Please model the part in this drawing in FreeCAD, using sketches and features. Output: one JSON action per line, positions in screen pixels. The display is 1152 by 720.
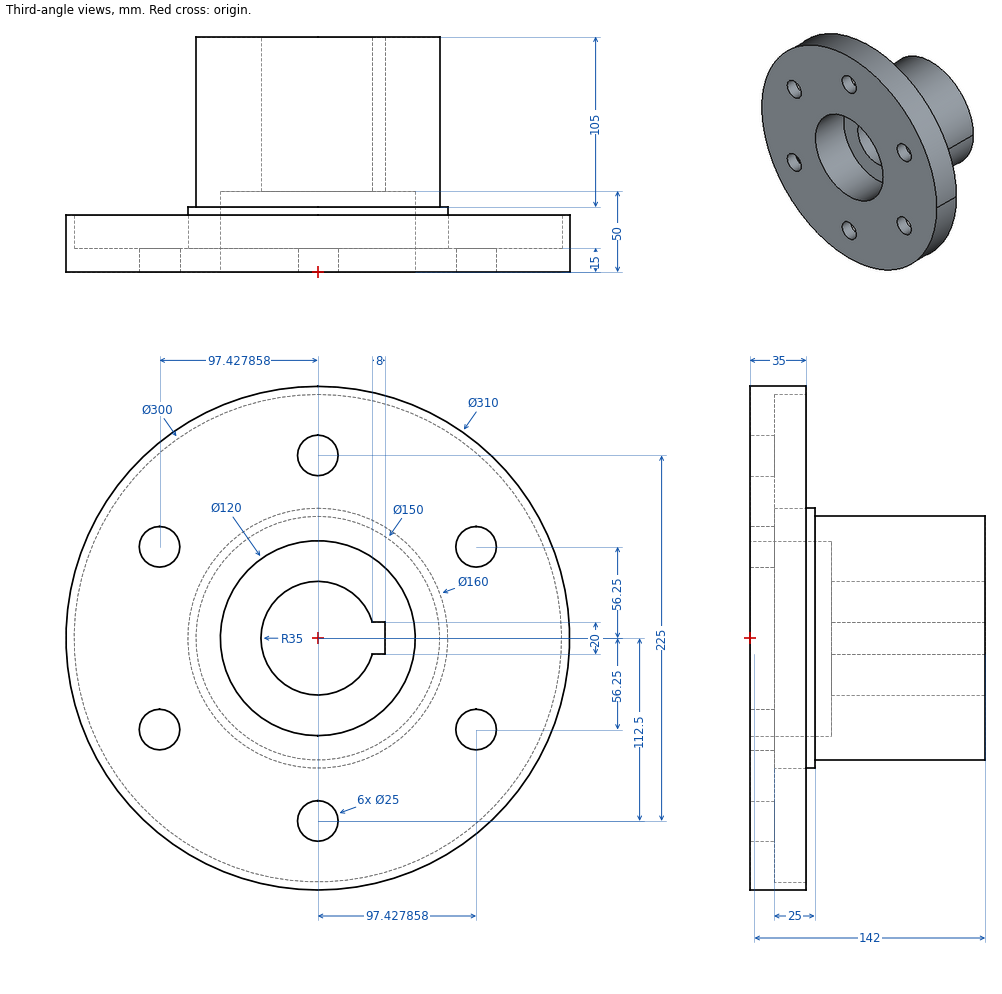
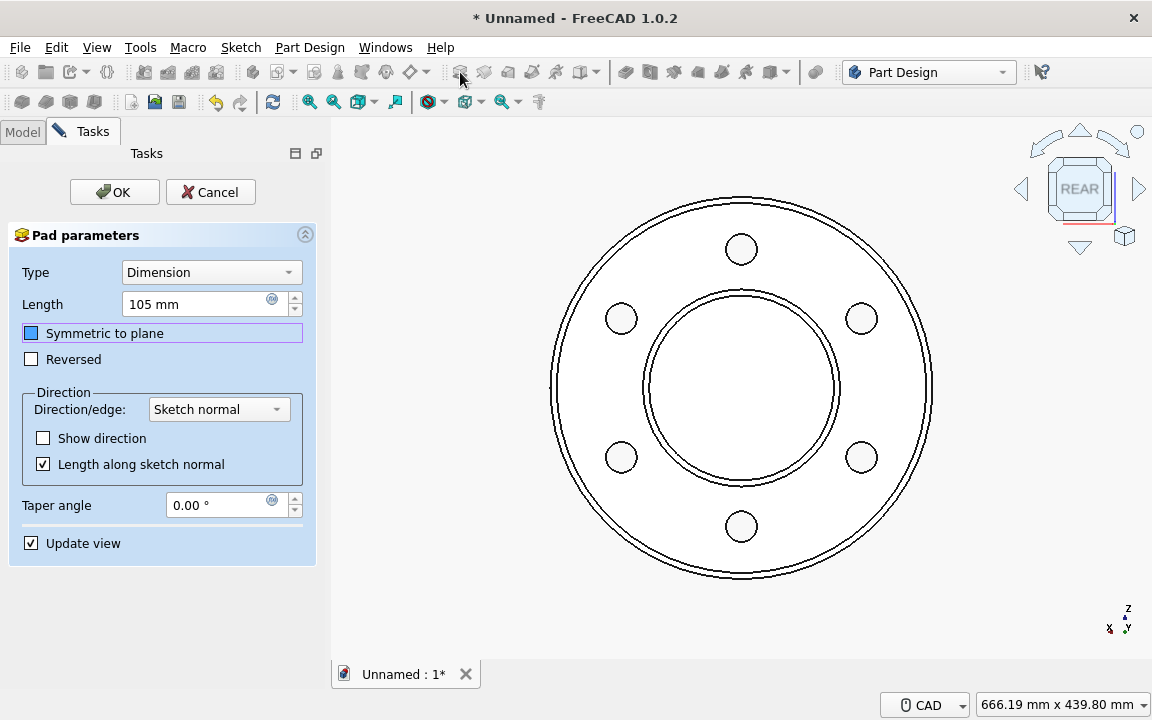
{"action": "left_click", "coordinate": [115, 192]}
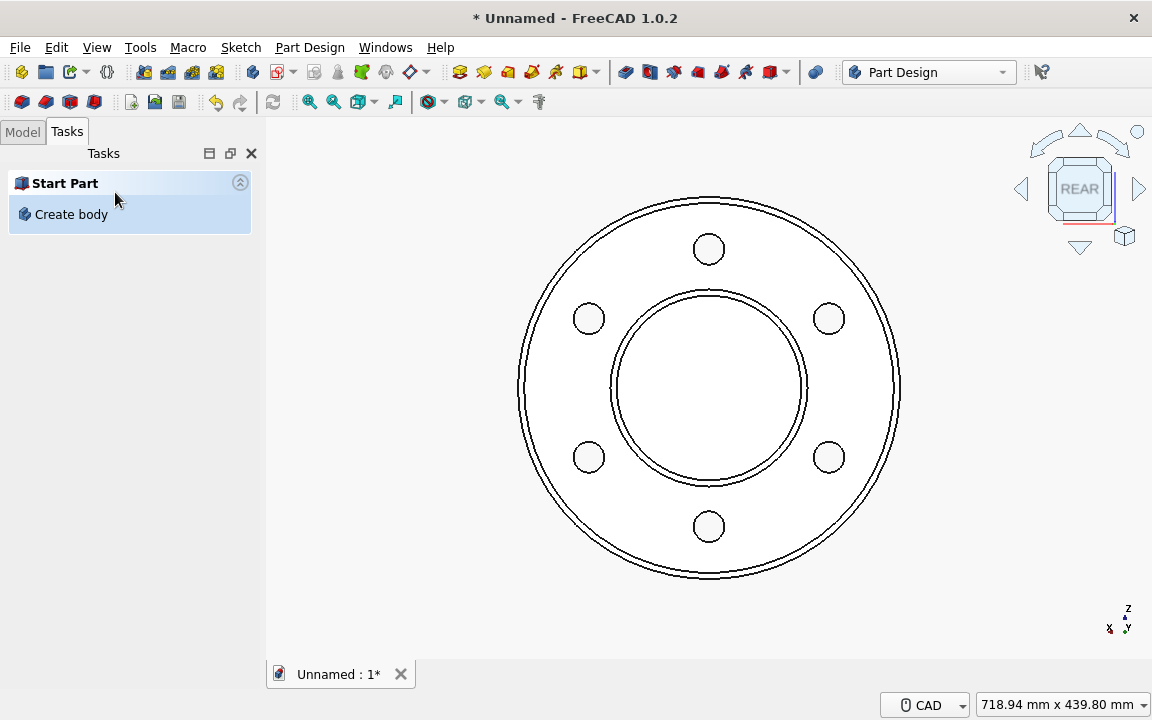
{"action": "left_click", "coordinate": [709, 387]}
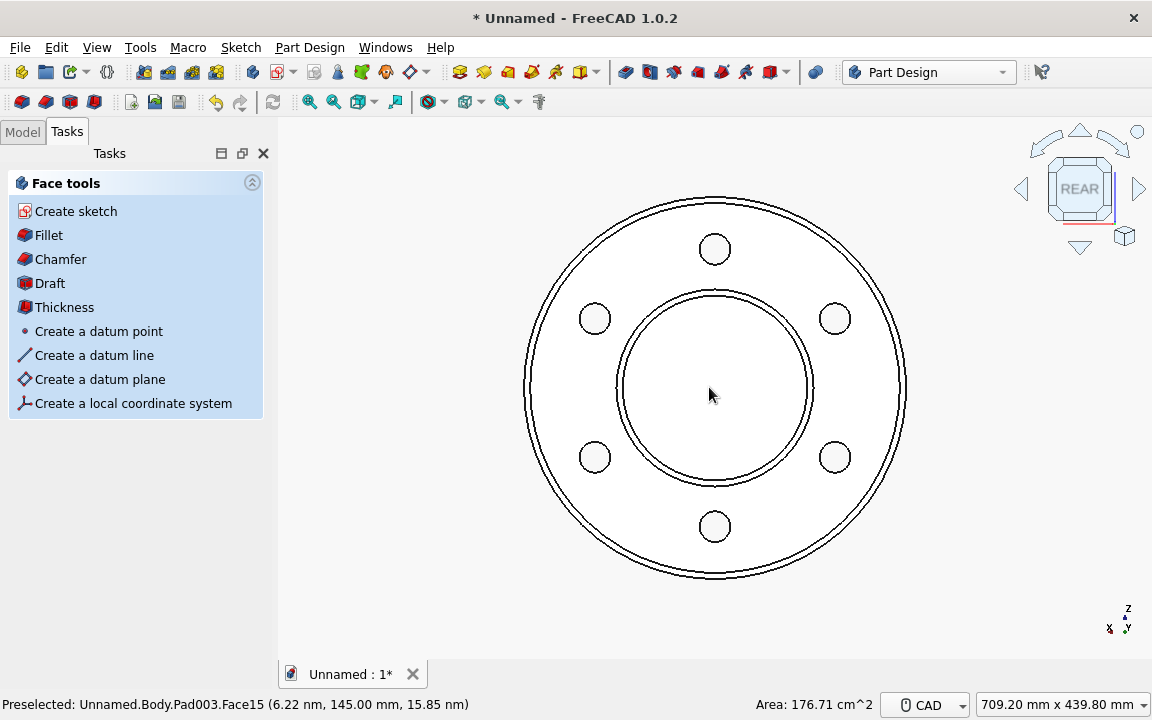
{"action": "left_click", "coordinate": [278, 72]}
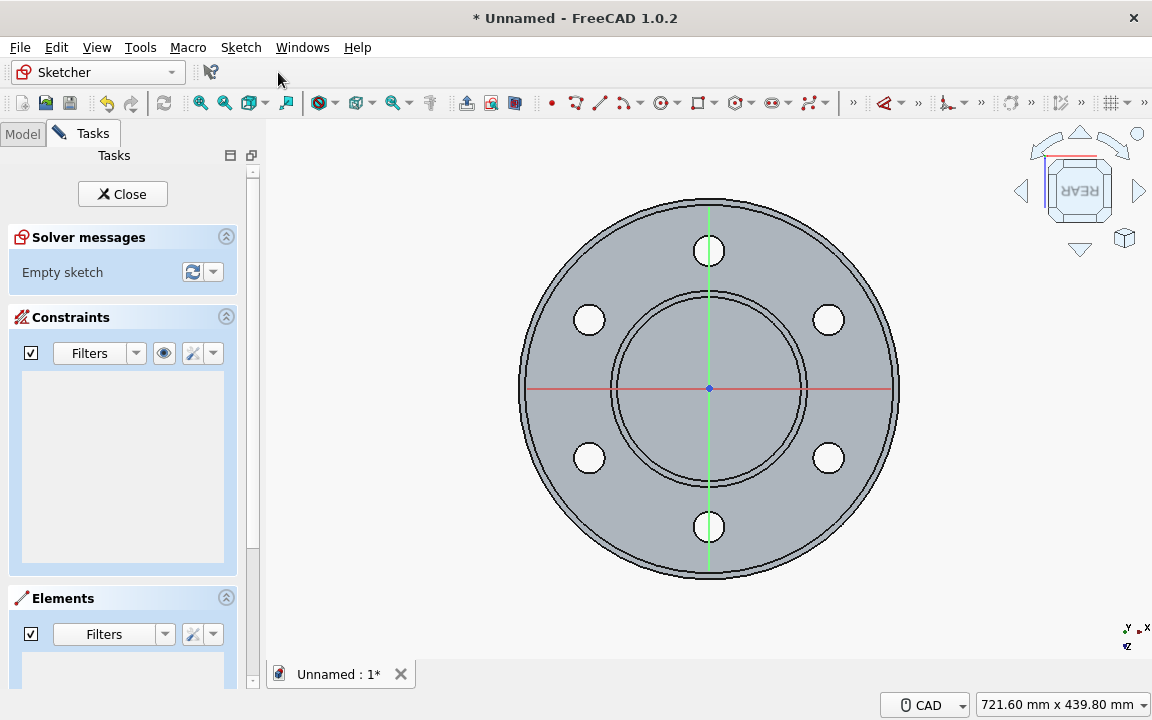
{"action": "scroll", "coordinate": [731, 389], "scroll_direction": "up", "scroll_amount": 8}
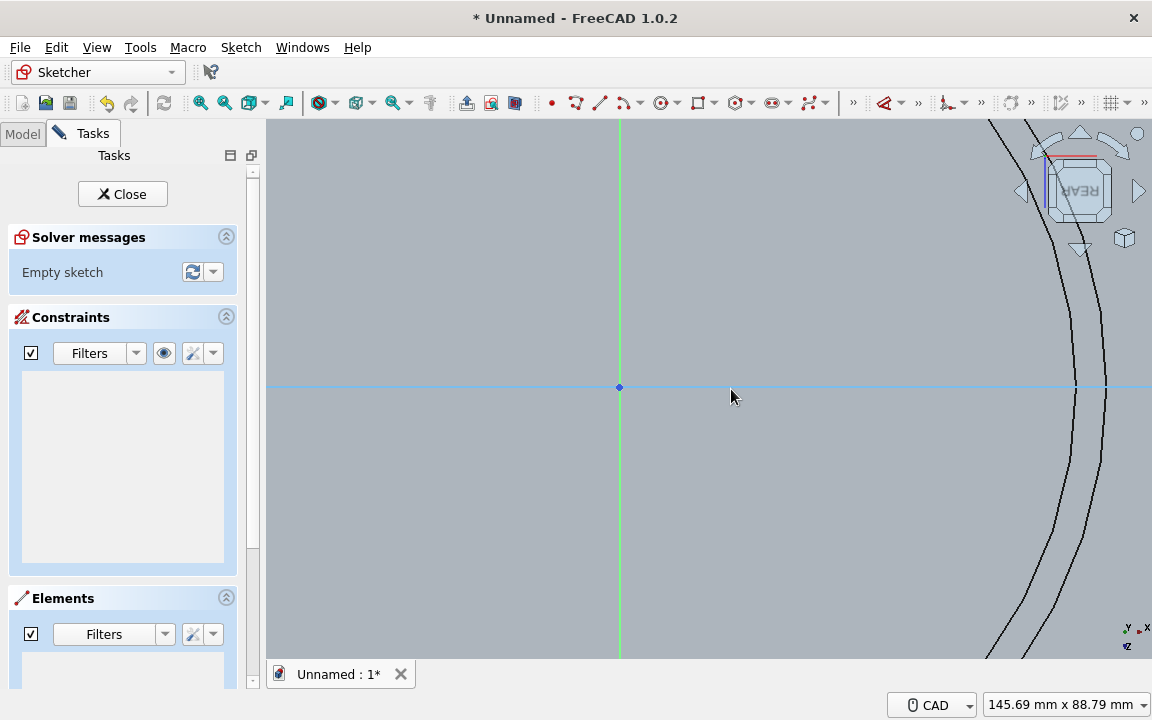
{"action": "left_click", "coordinate": [576, 104]}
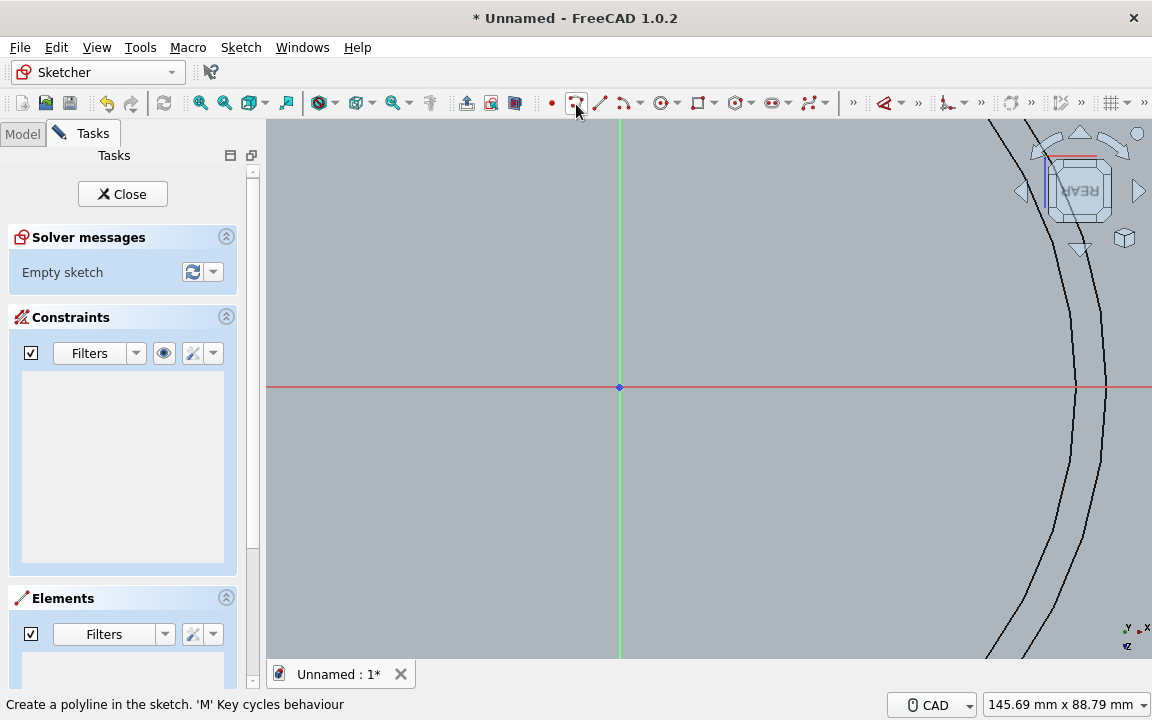
{"action": "left_click", "coordinate": [824, 448]}
{"action": "left_click", "coordinate": [873, 448]}
{"action": "left_click", "coordinate": [873, 326]}
{"action": "left_click", "coordinate": [824, 326]}
{"action": "right_click", "coordinate": [824, 326]}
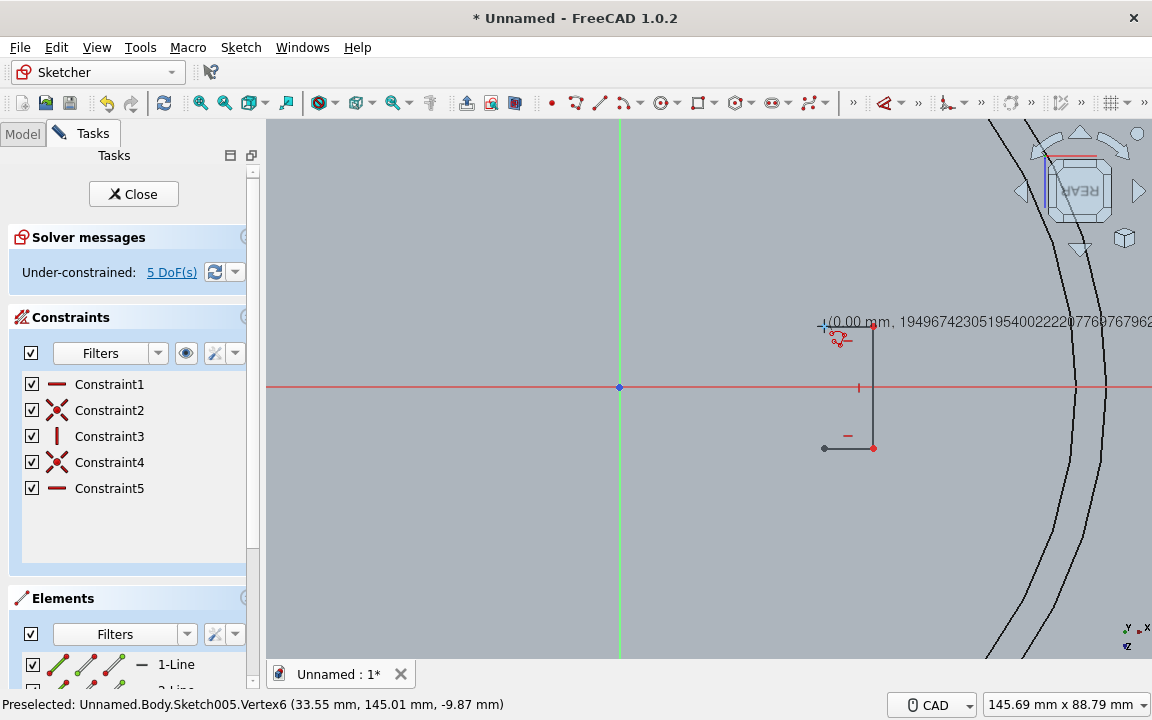
{"action": "left_click", "coordinate": [642, 104]}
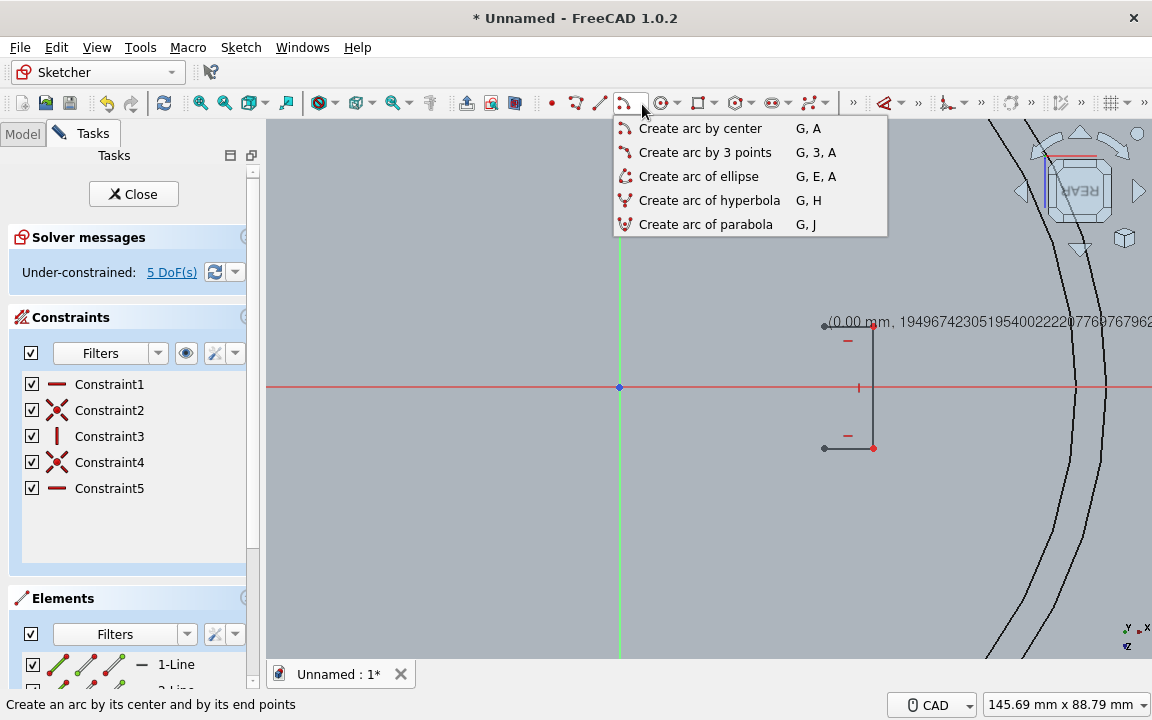
{"action": "left_click", "coordinate": [750, 152]}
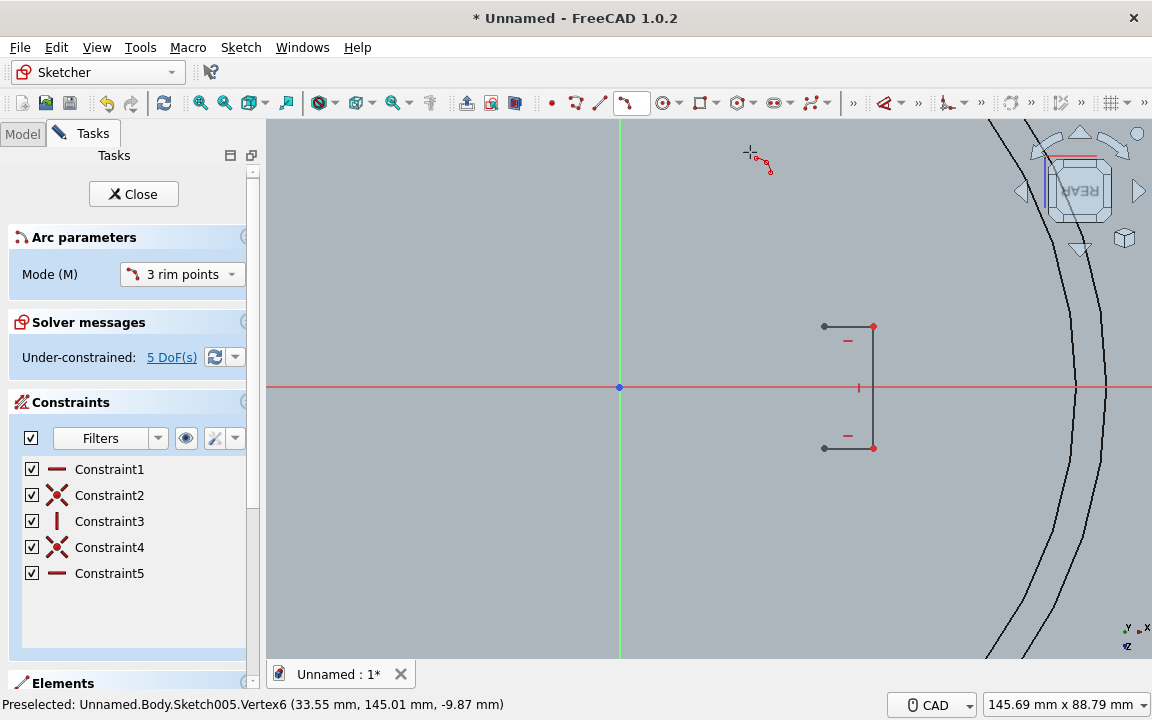
{"action": "left_click", "coordinate": [824, 327]}
{"action": "left_click", "coordinate": [824, 449]}
{"action": "left_click", "coordinate": [441, 272]}
{"action": "key", "text": "Escape"}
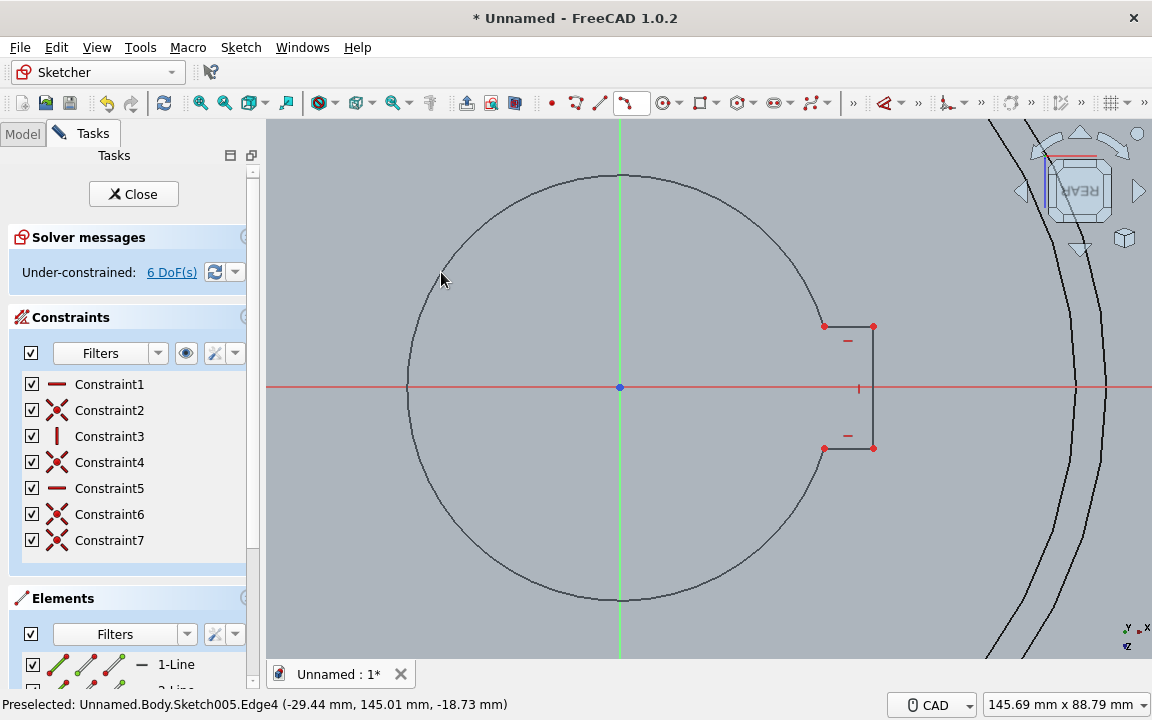
{"action": "left_click_drag", "start_coordinate": [610, 377], "coordinate": [630, 398]}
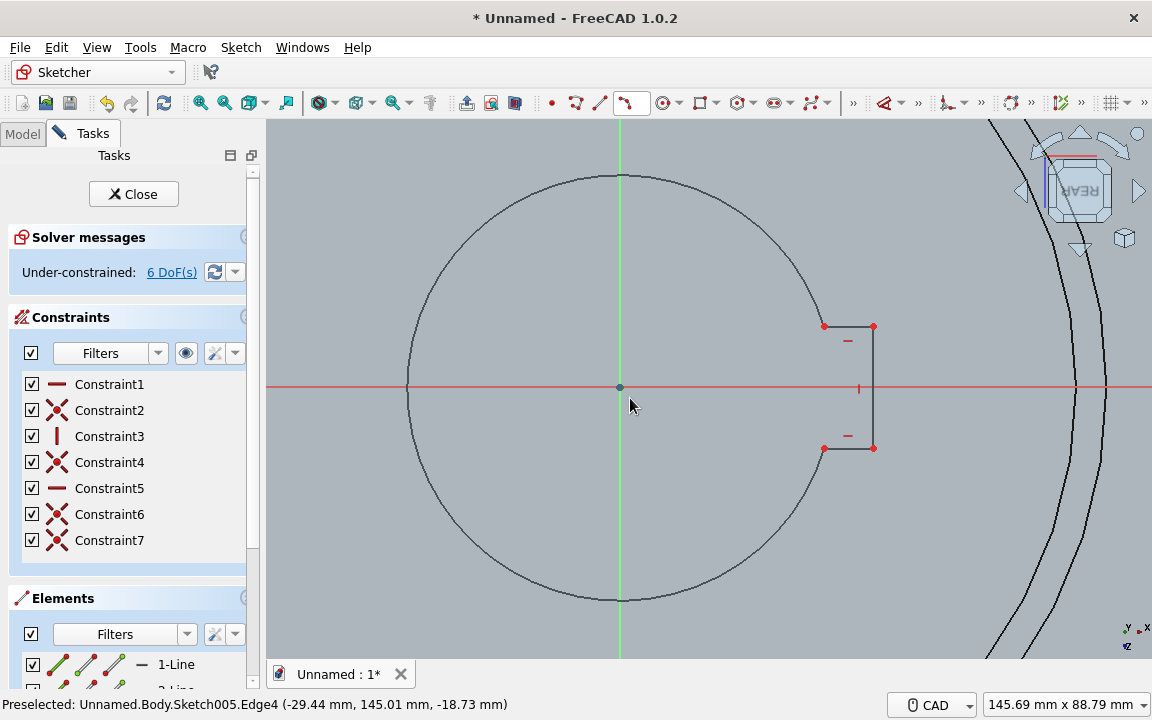
{"action": "key", "text": "c"}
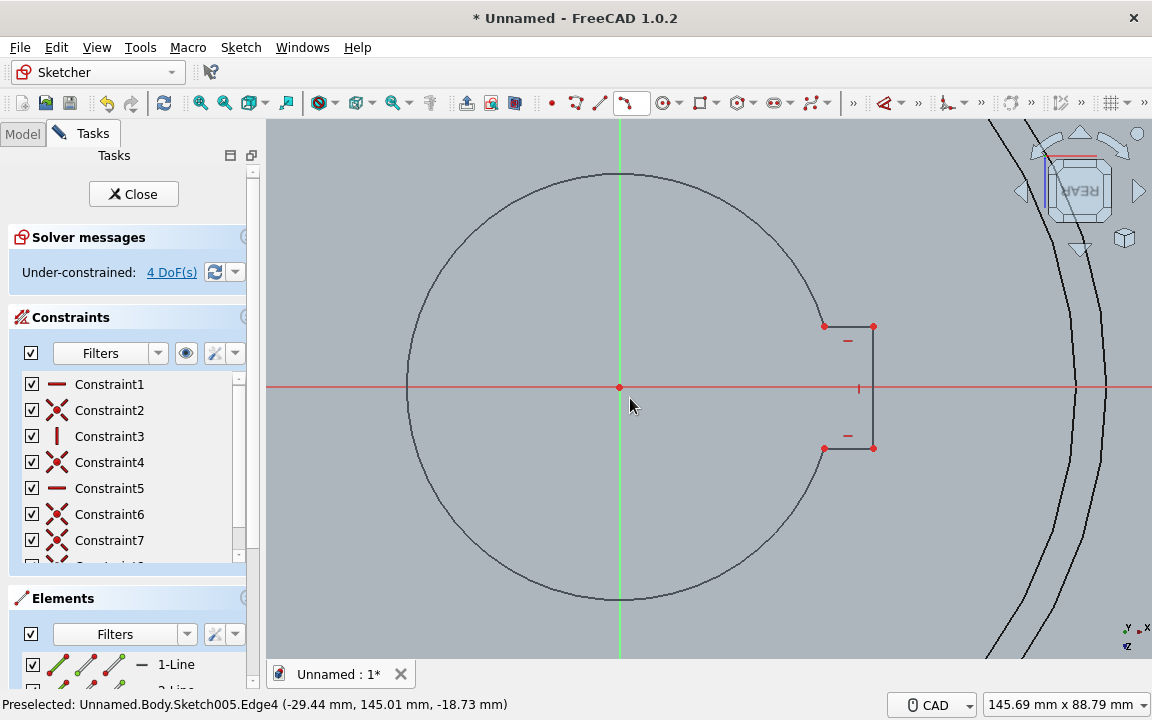
{"action": "left_click", "coordinate": [884, 104]}